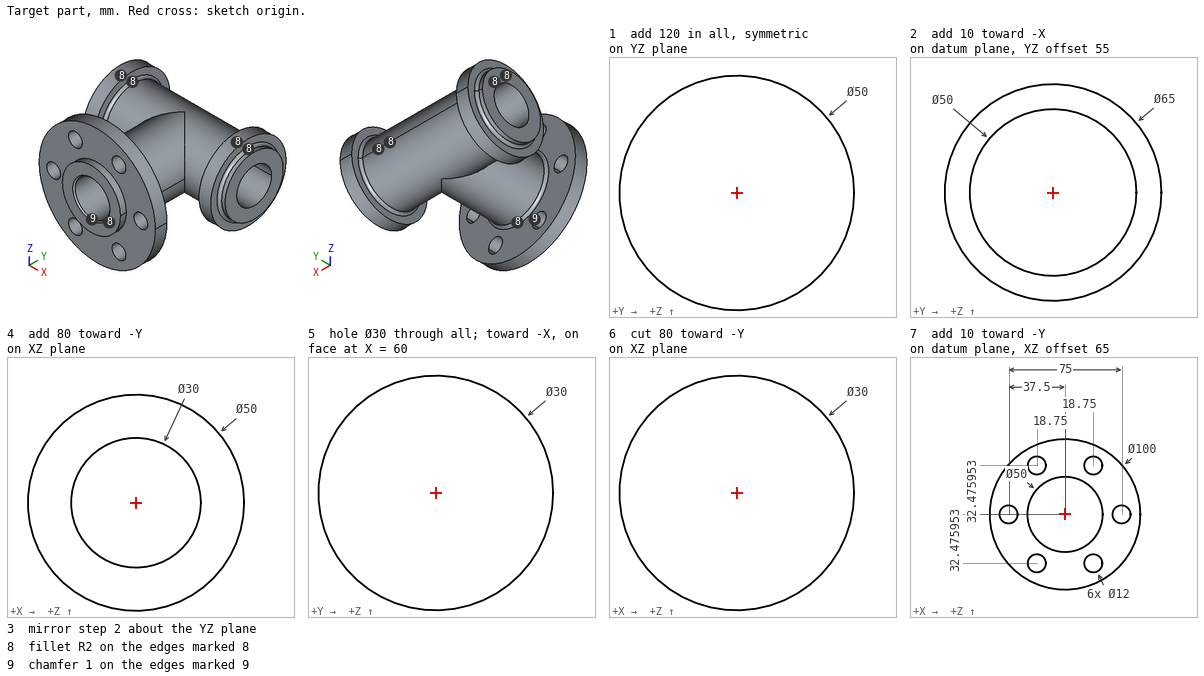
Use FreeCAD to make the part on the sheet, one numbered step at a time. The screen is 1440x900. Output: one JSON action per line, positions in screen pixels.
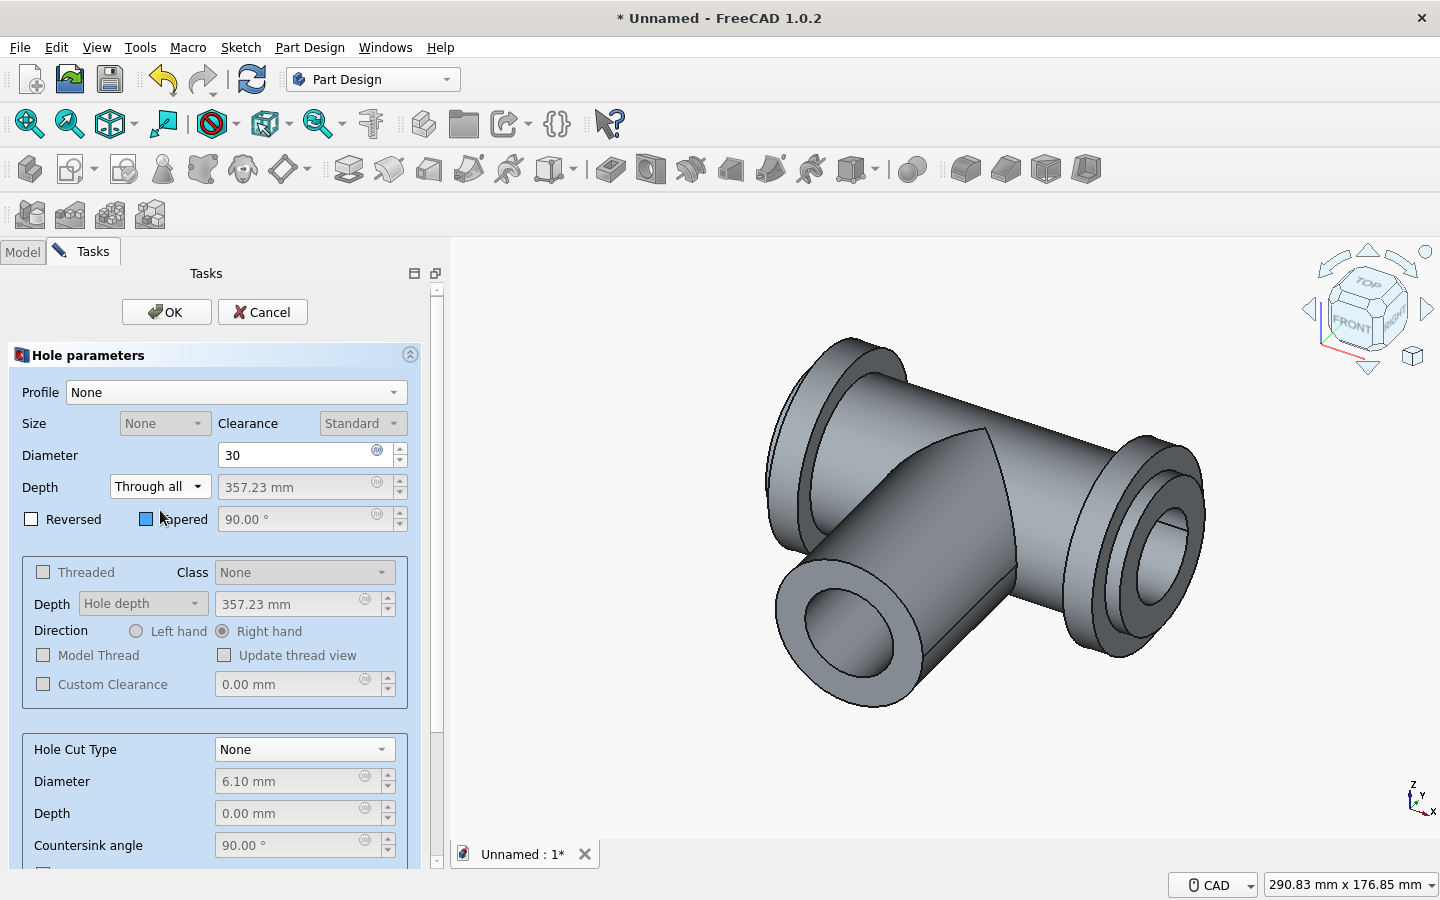
{"action": "left_click", "coordinate": [167, 312]}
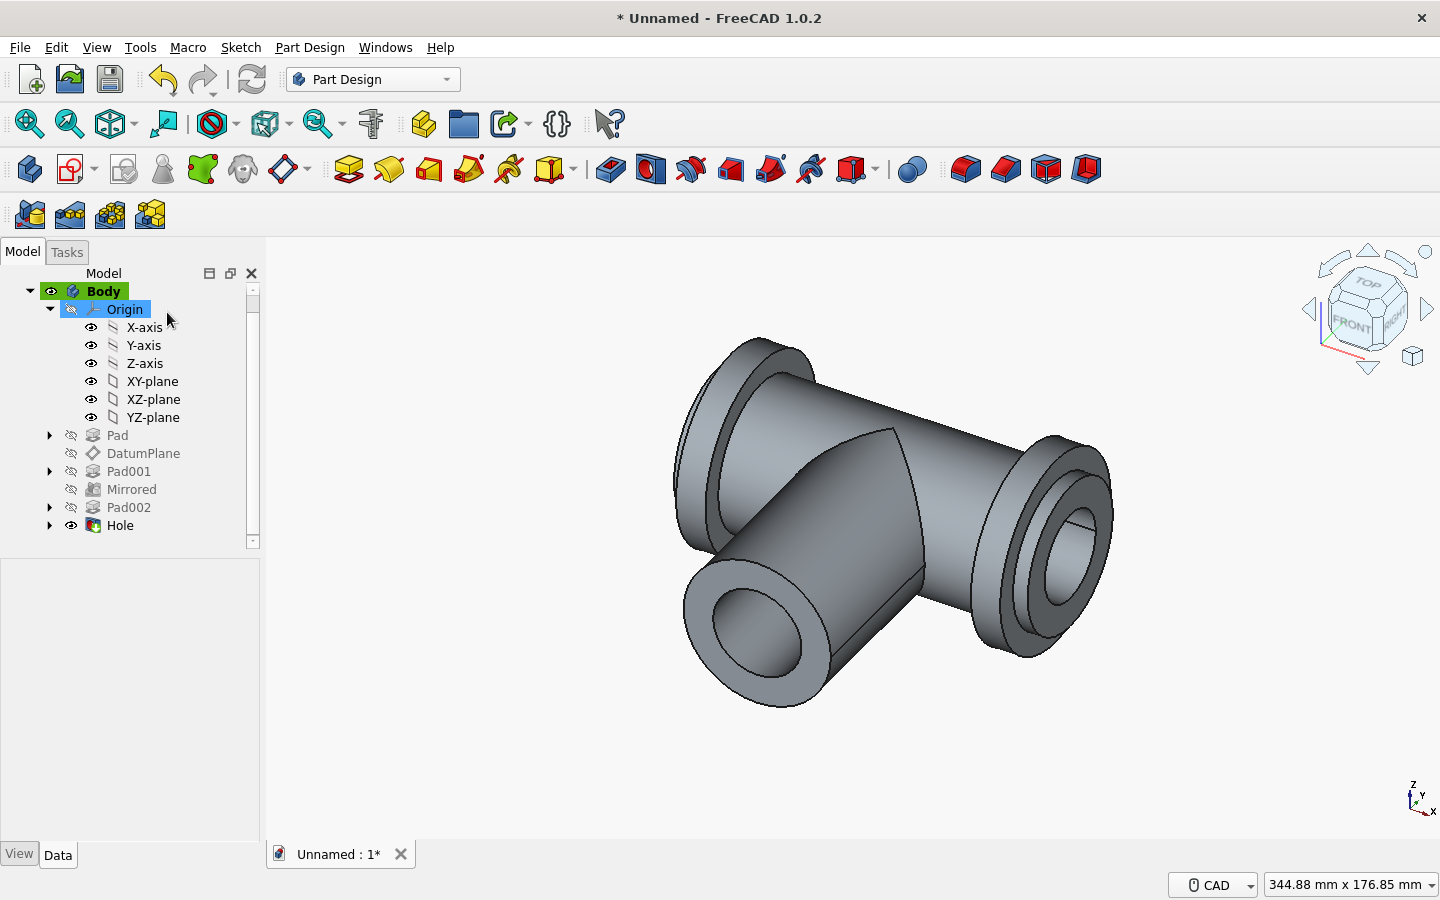
{"action": "left_click", "coordinate": [70, 170]}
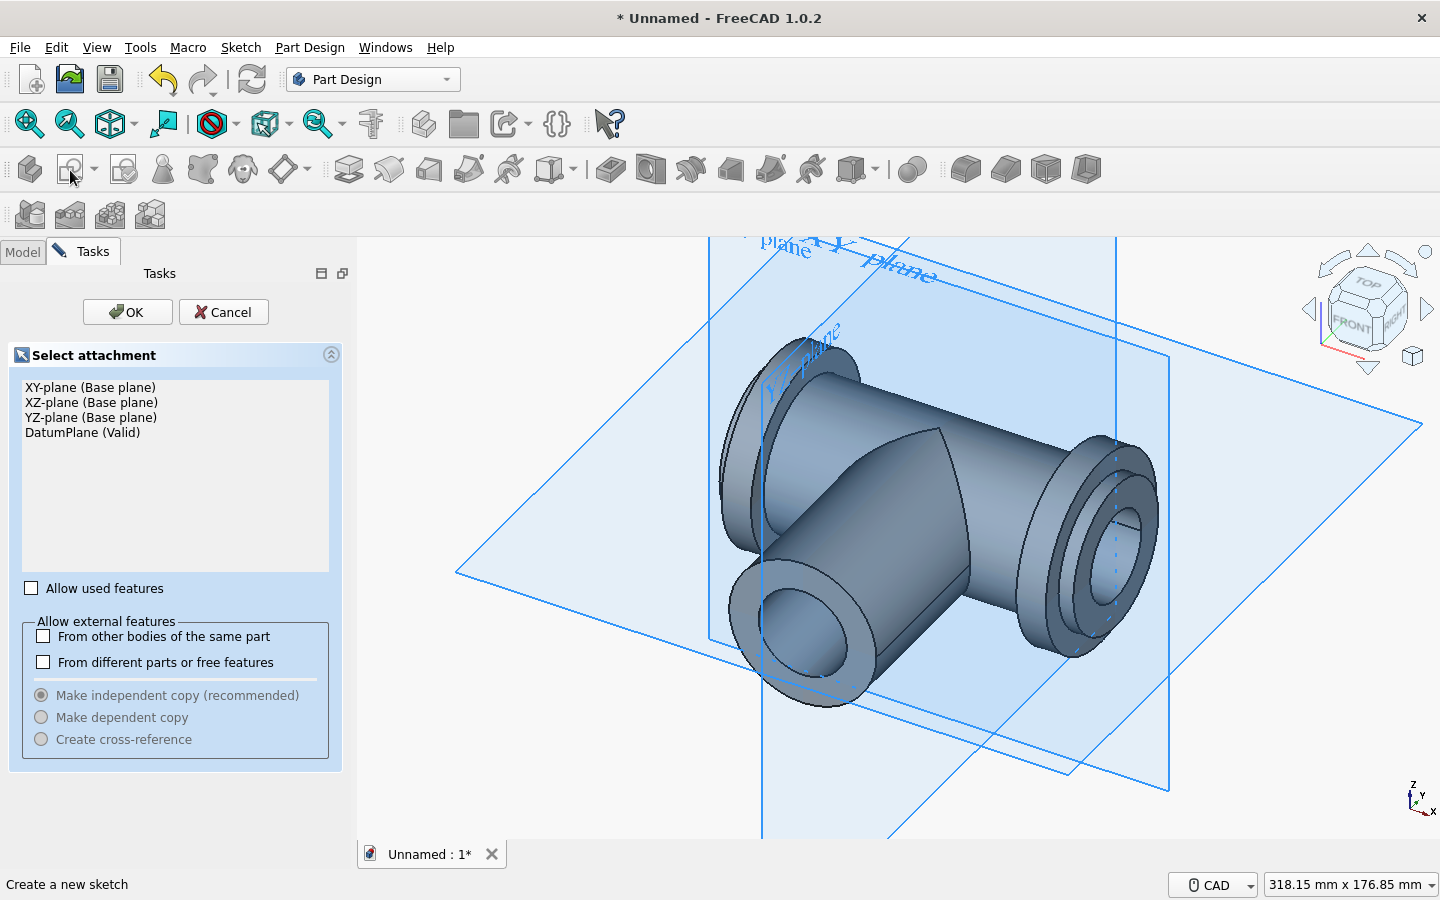
{"action": "left_click", "coordinate": [82, 402]}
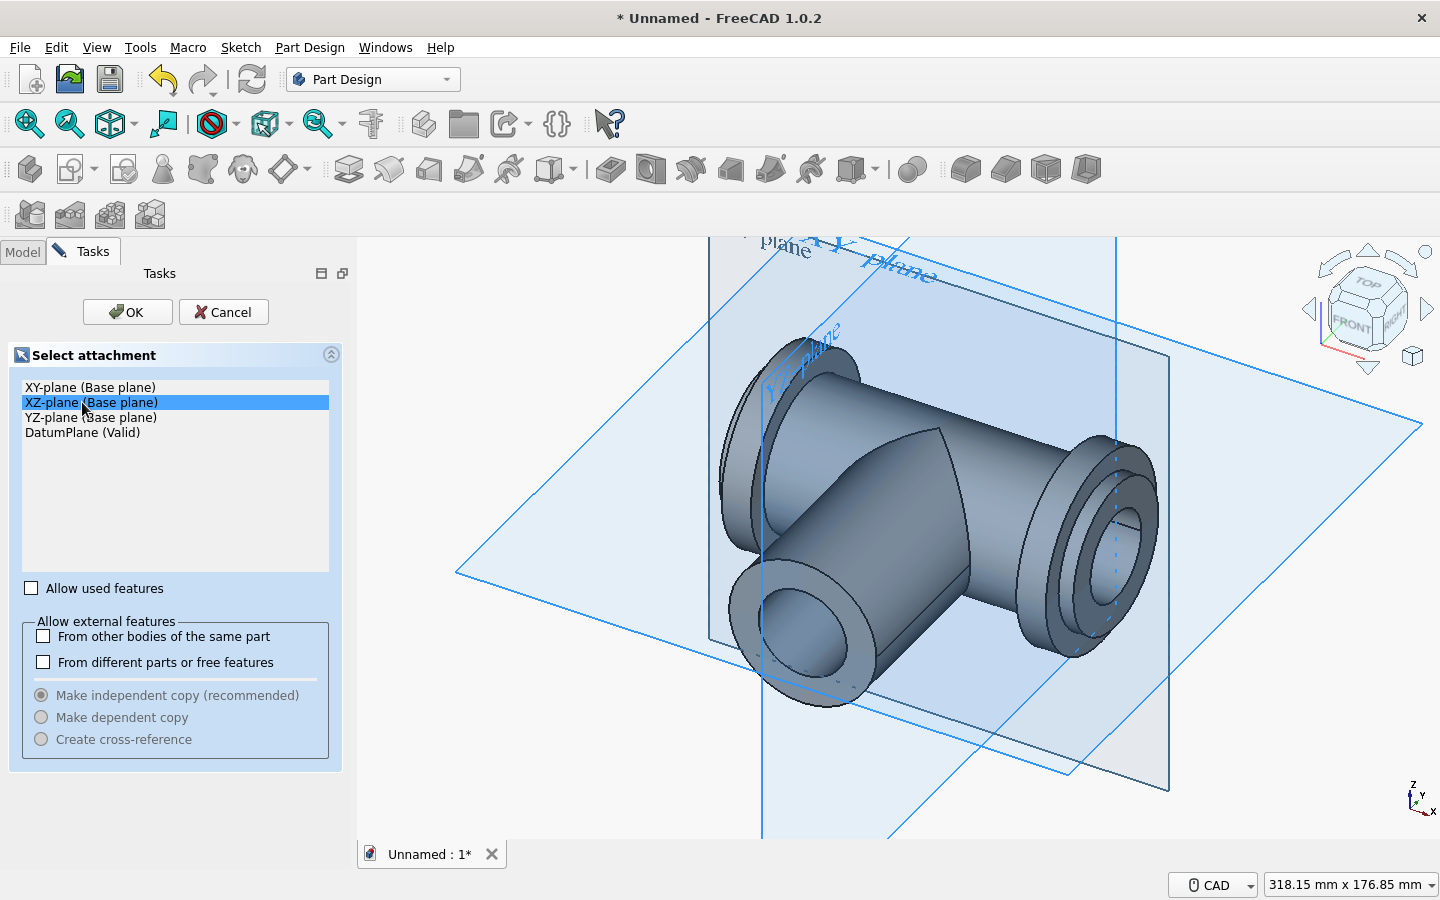
{"action": "left_click", "coordinate": [128, 312]}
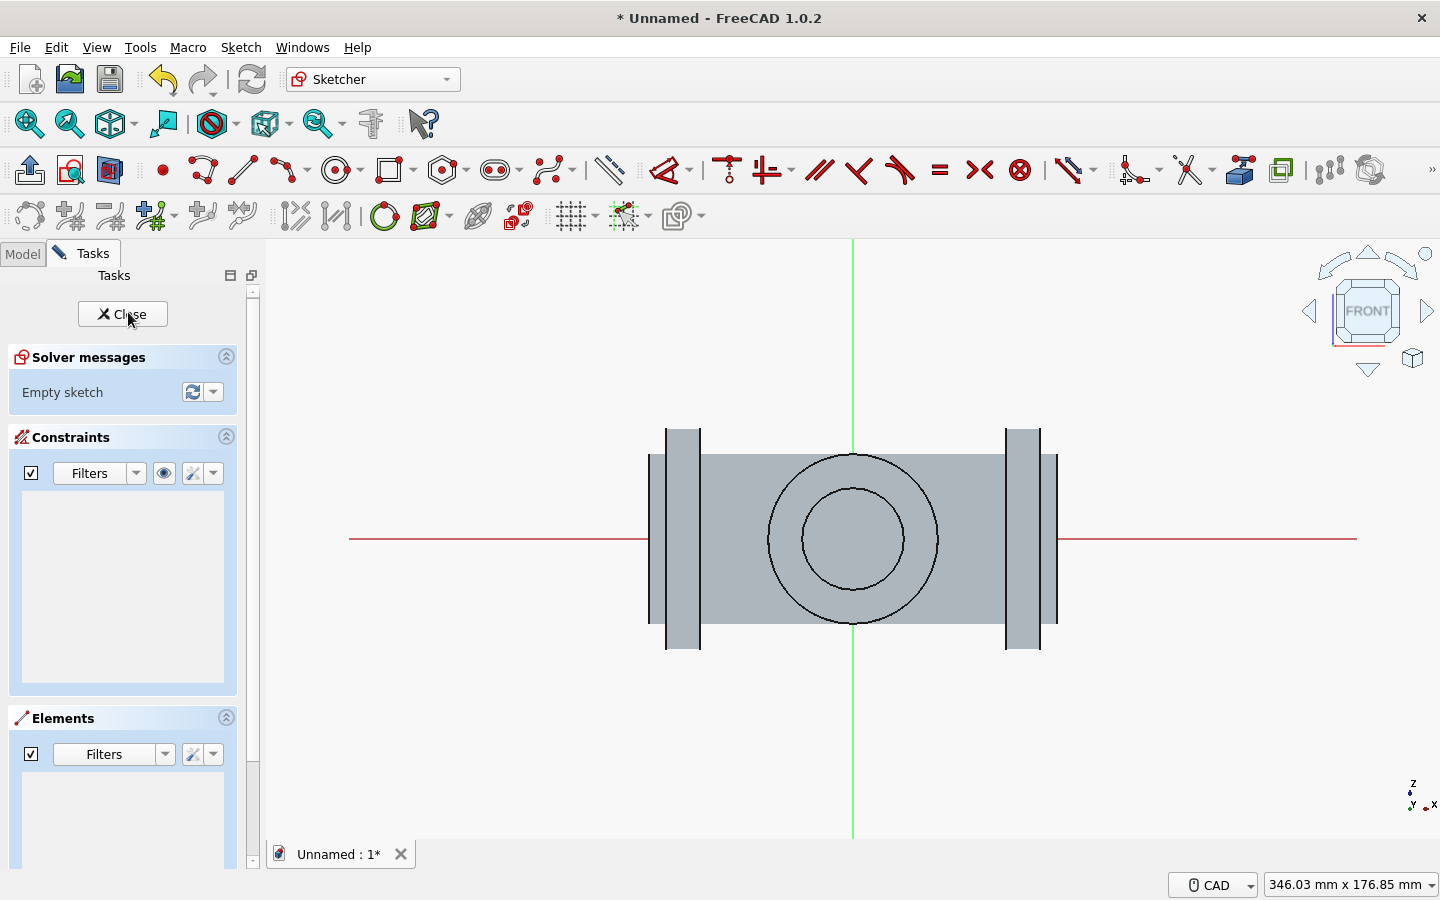
{"action": "key", "text": "q s"}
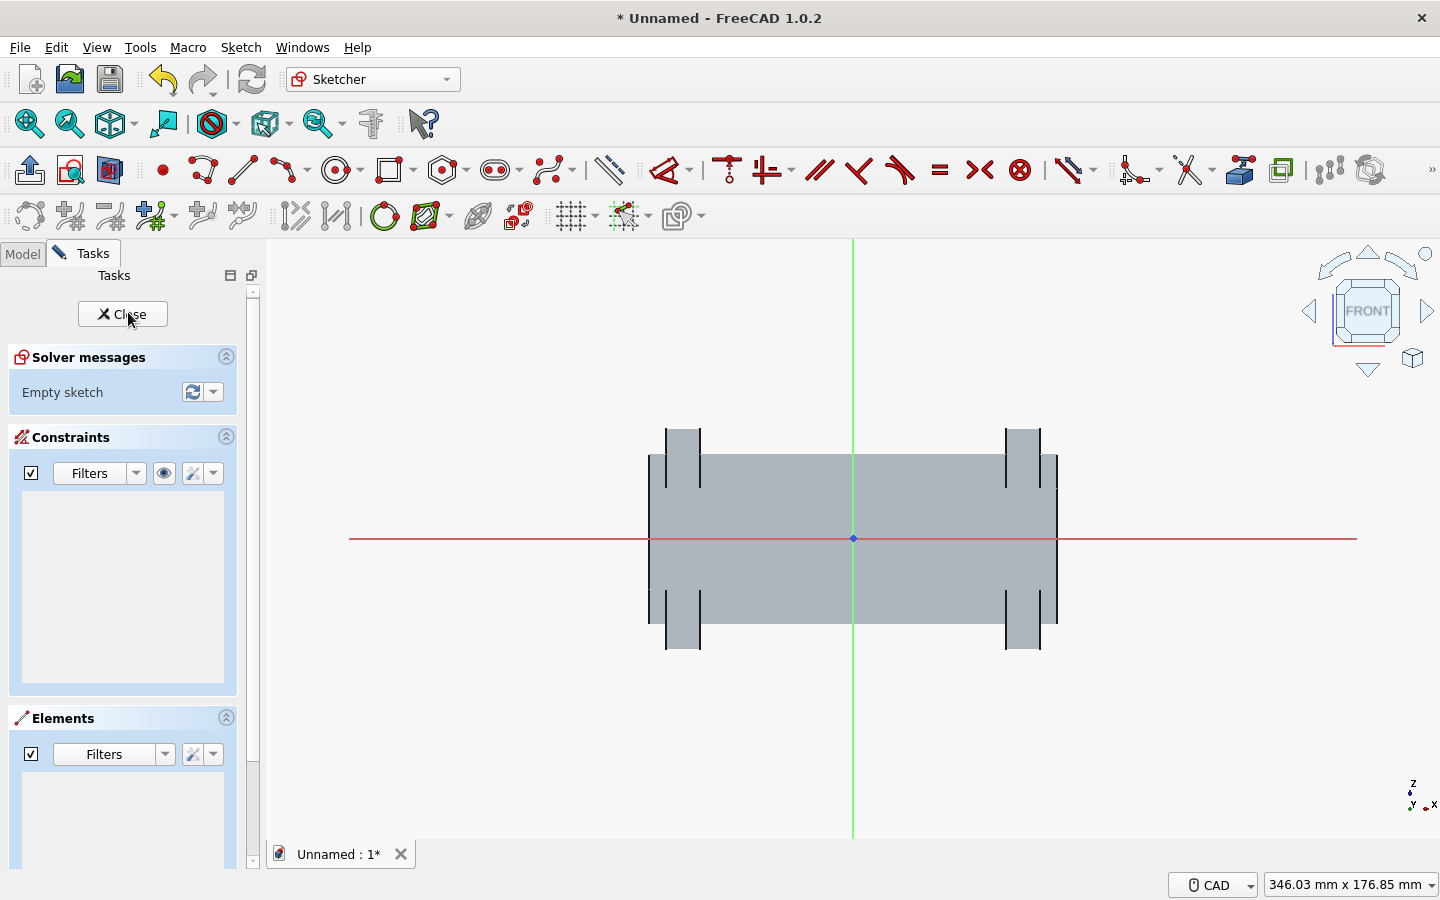
{"action": "scroll", "coordinate": [875, 539], "scroll_direction": "up", "scroll_amount": 7}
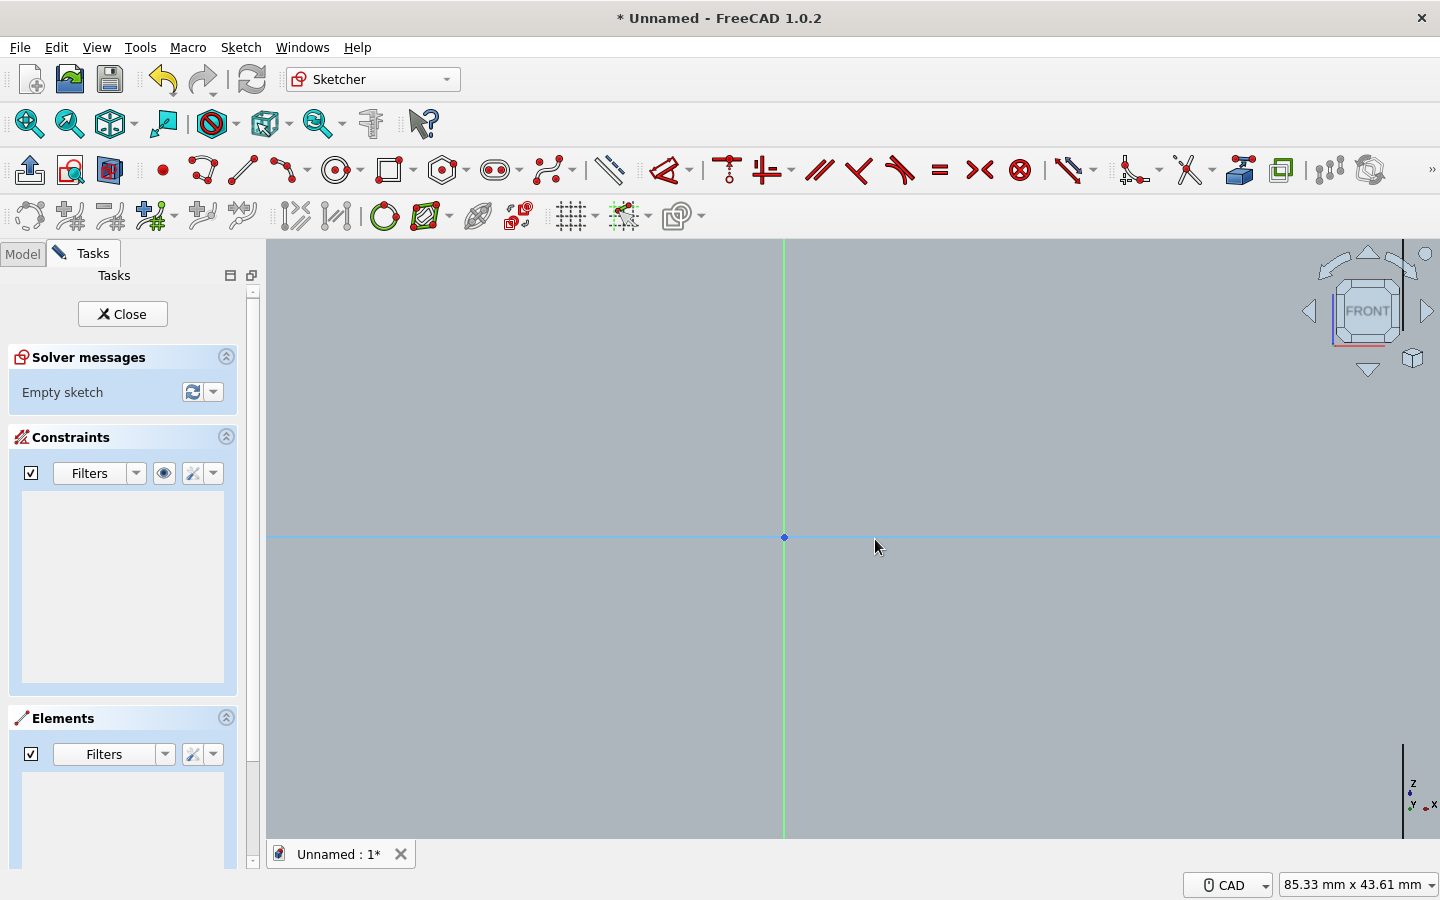
{"action": "key", "text": "g c"}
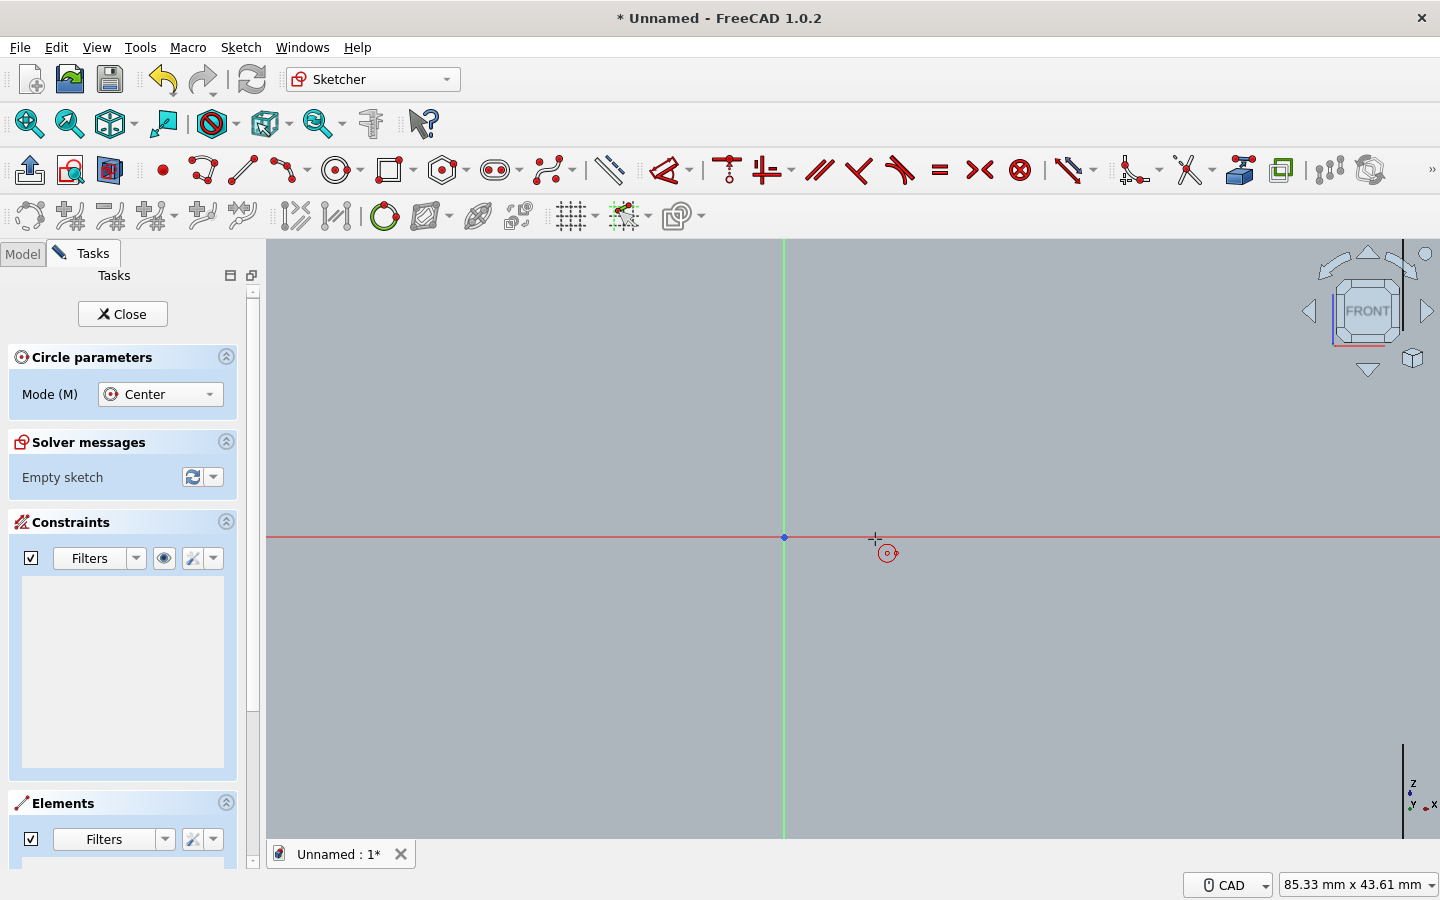
{"action": "left_click", "coordinate": [784, 537]}
{"action": "left_click", "coordinate": [930, 392]}
{"action": "key", "text": "Escape"}